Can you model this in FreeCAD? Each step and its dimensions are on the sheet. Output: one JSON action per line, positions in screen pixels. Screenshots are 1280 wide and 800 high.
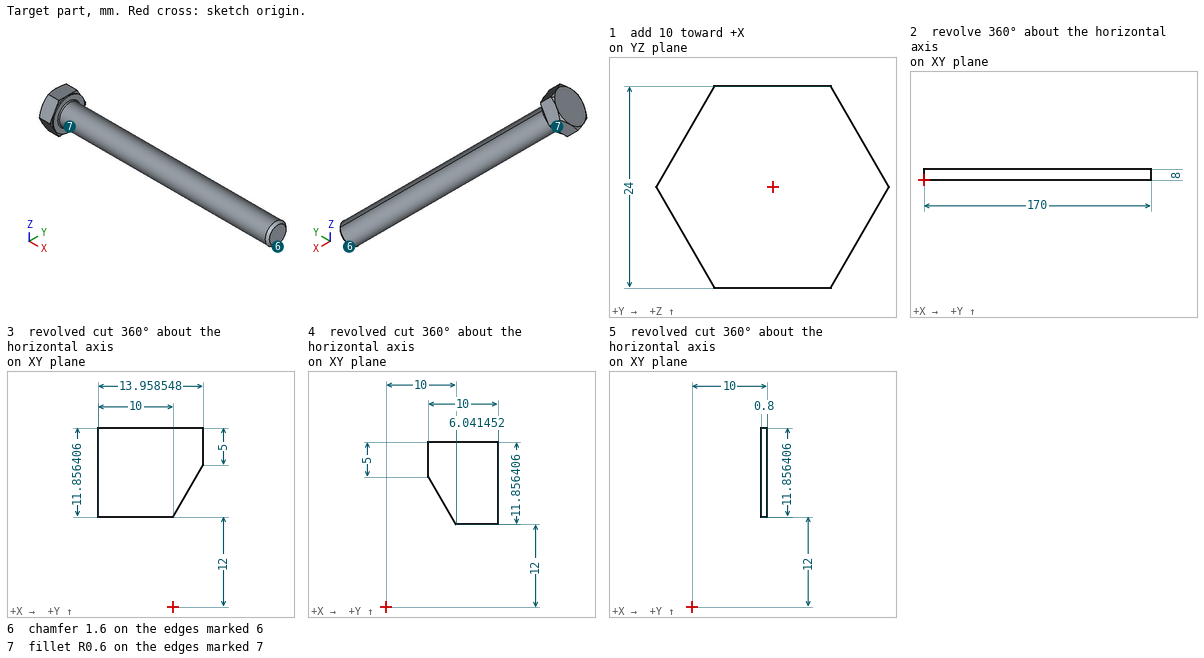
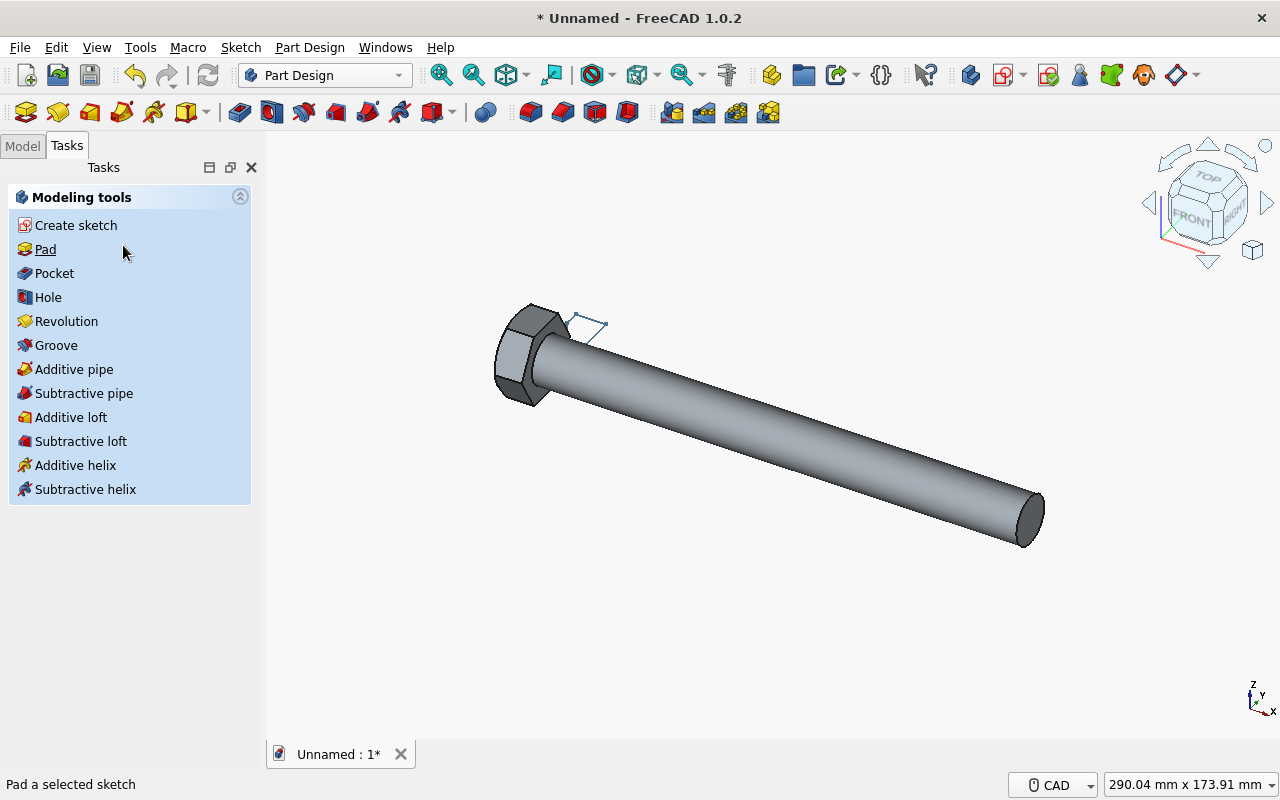
{"action": "left_click", "coordinate": [304, 112]}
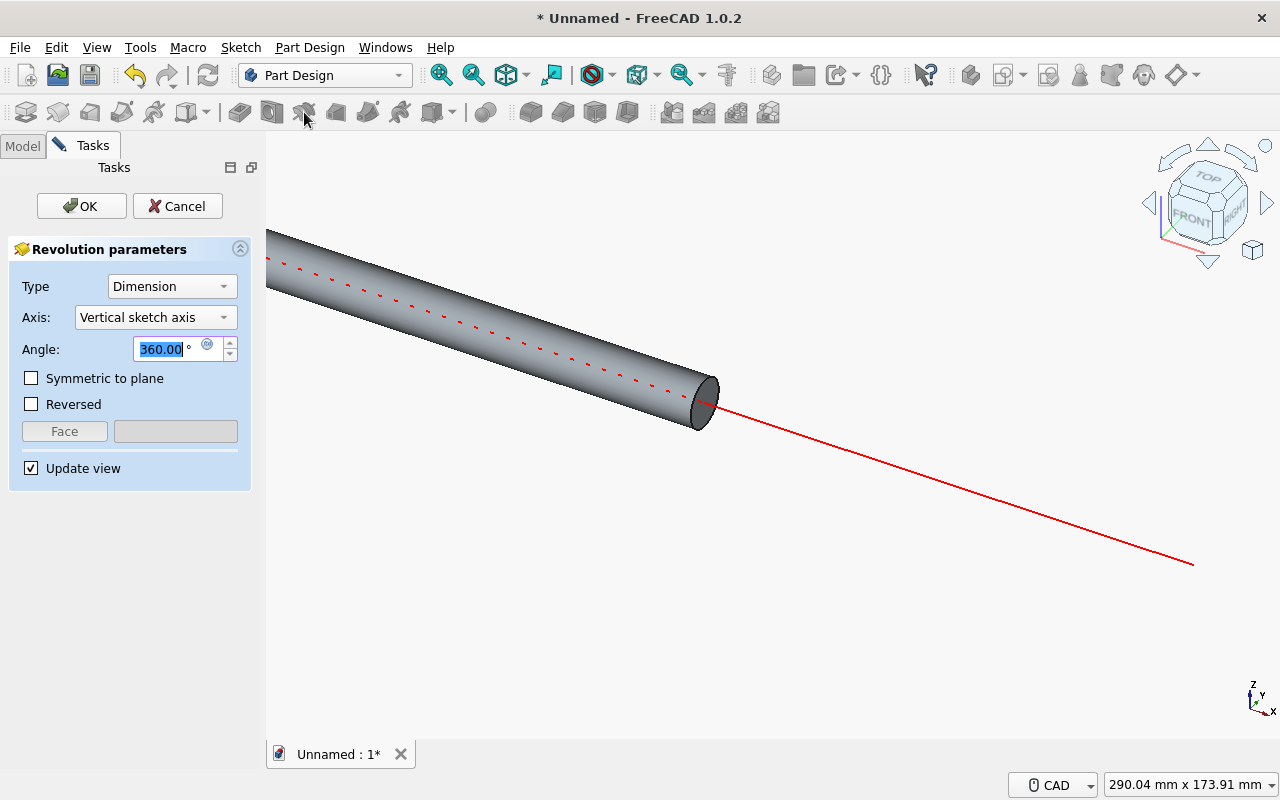
{"action": "left_click", "coordinate": [156, 318]}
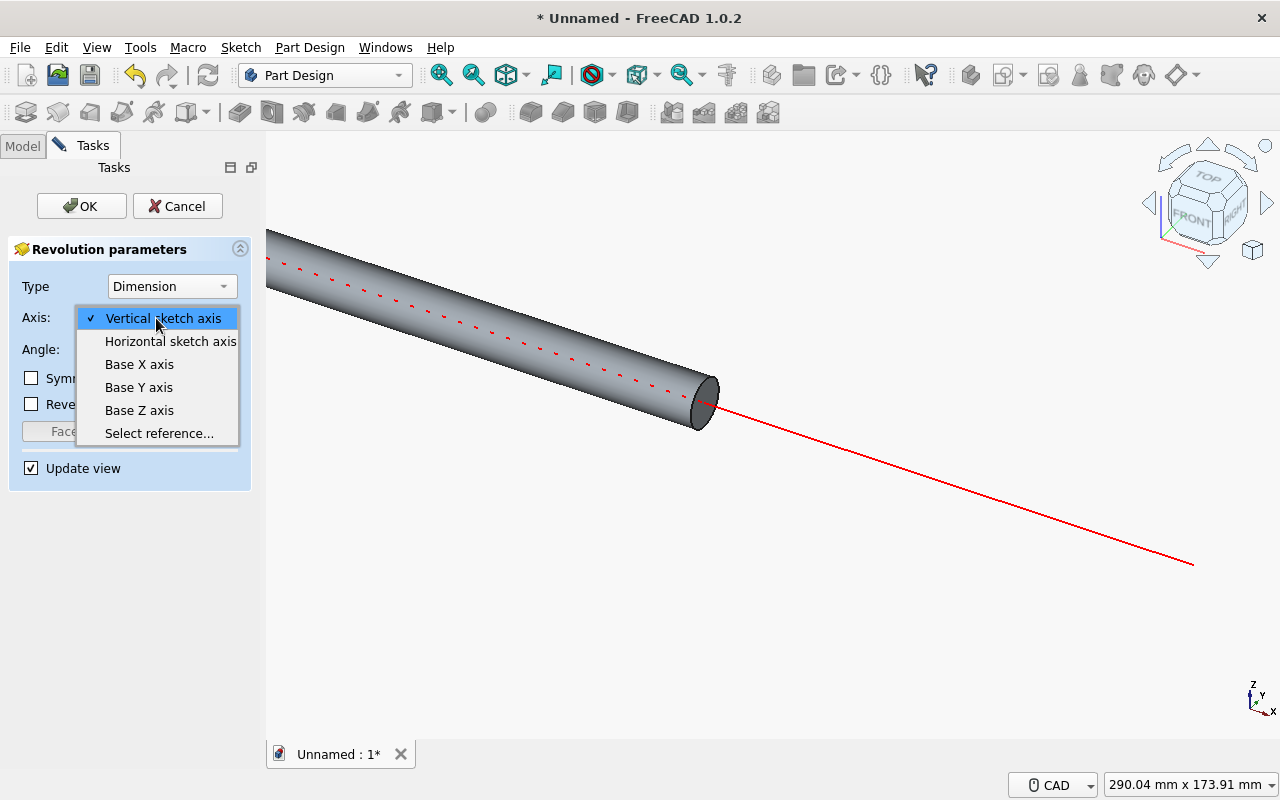
{"action": "left_click", "coordinate": [156, 342]}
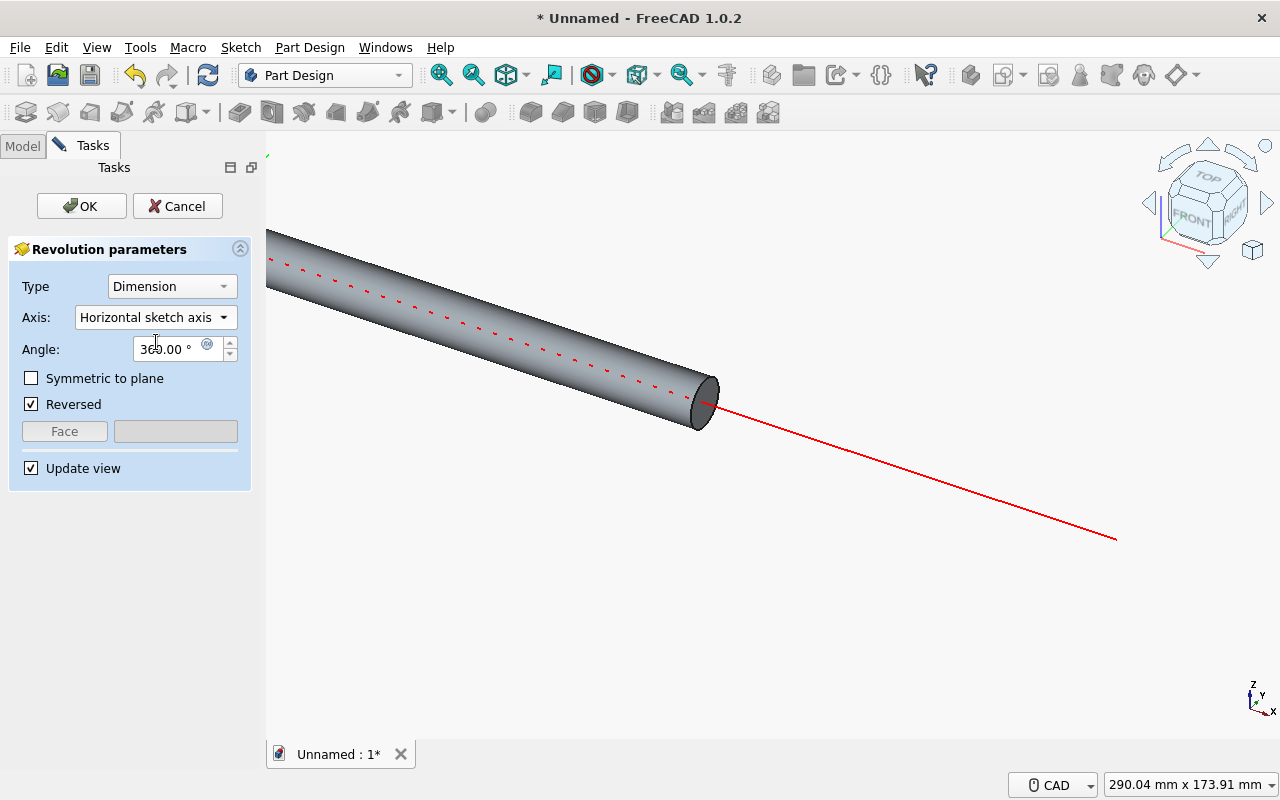
{"action": "left_click", "coordinate": [82, 206]}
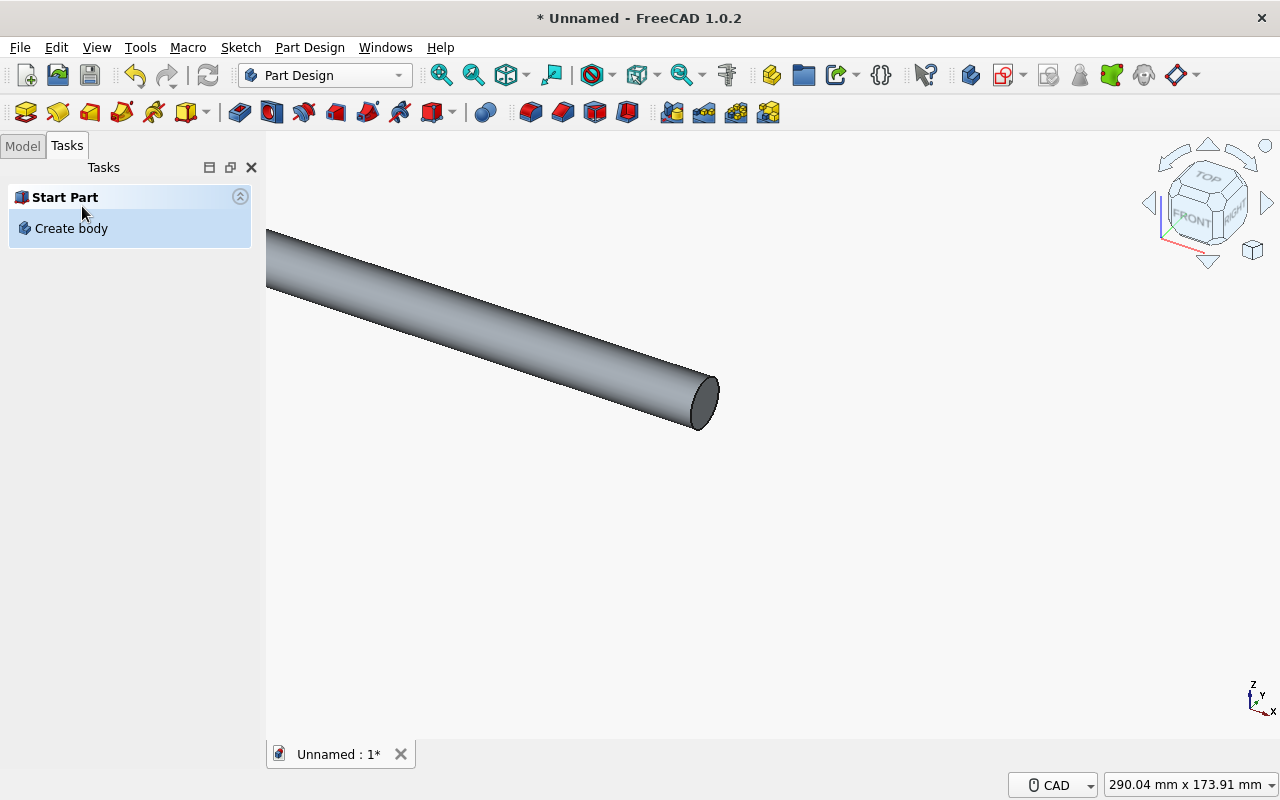
{"action": "left_click", "coordinate": [442, 76]}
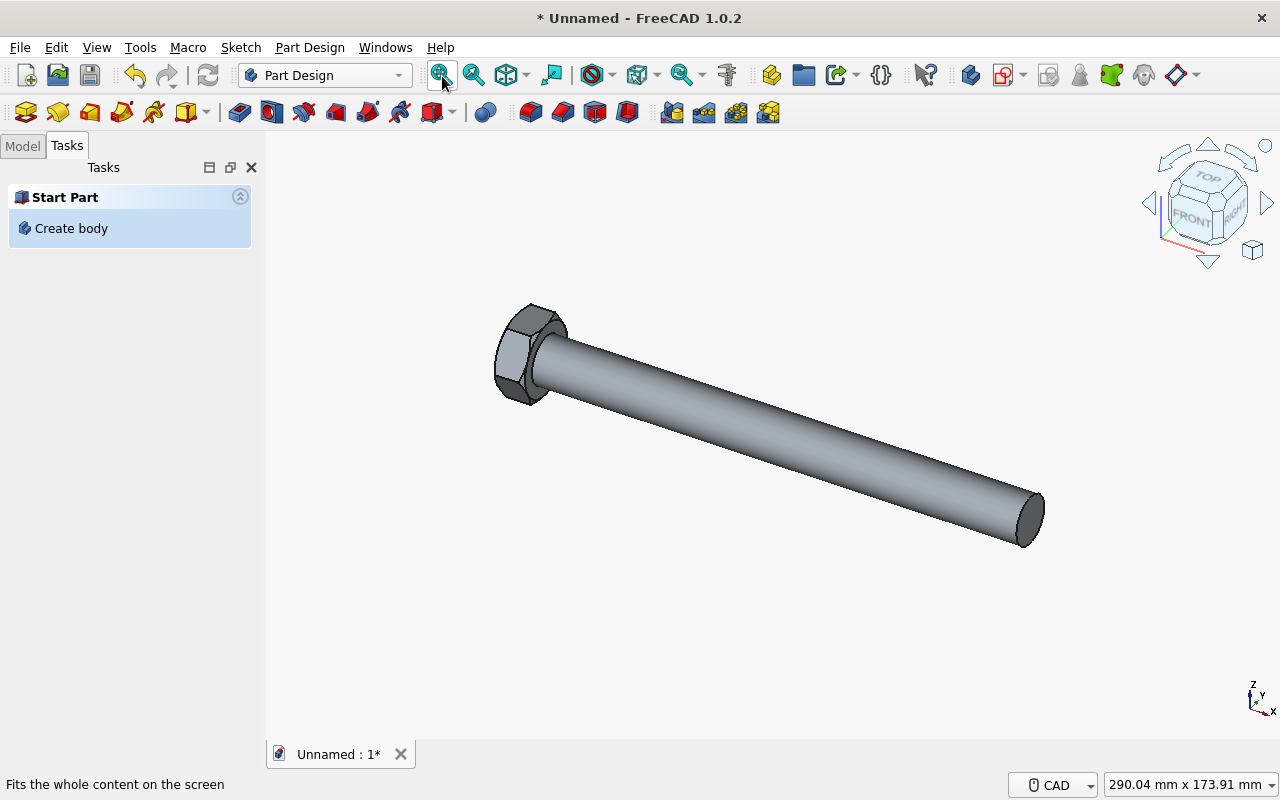
{"action": "left_click", "coordinate": [1004, 76]}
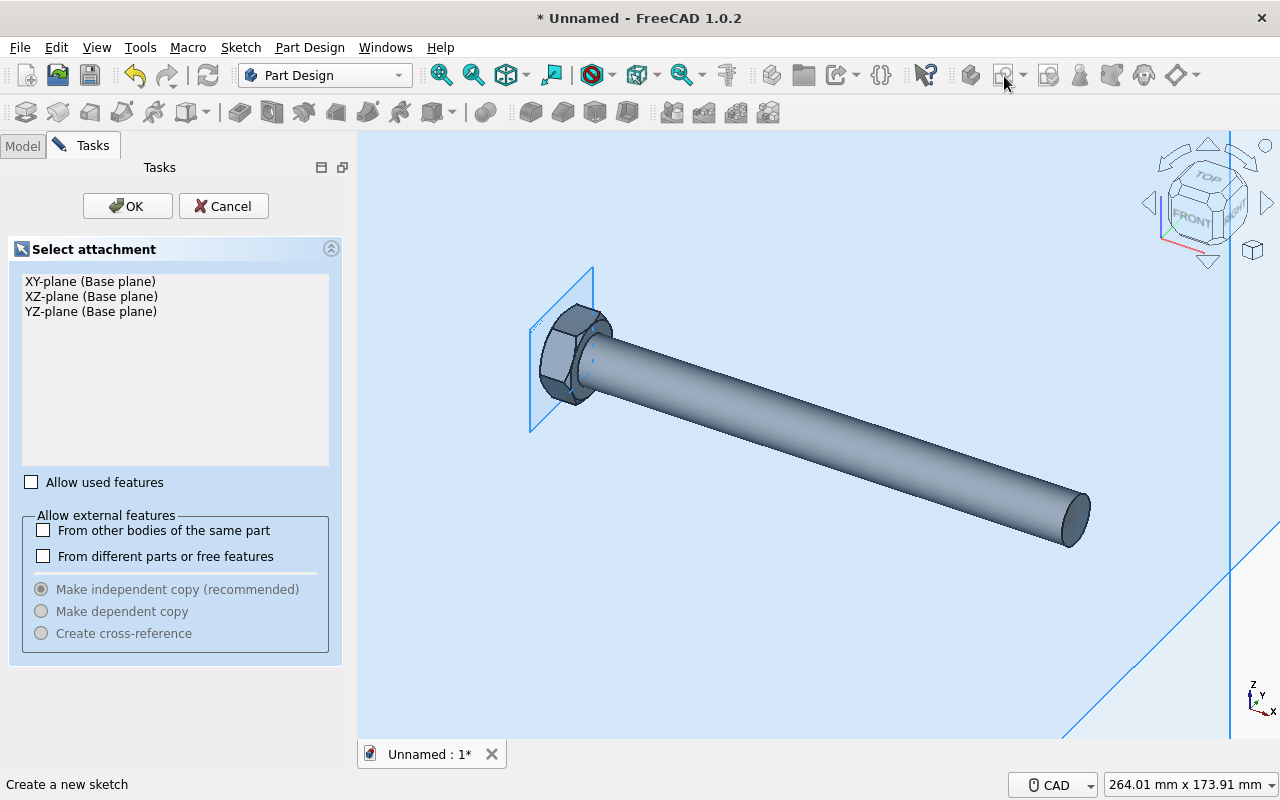
{"action": "left_click", "coordinate": [82, 282]}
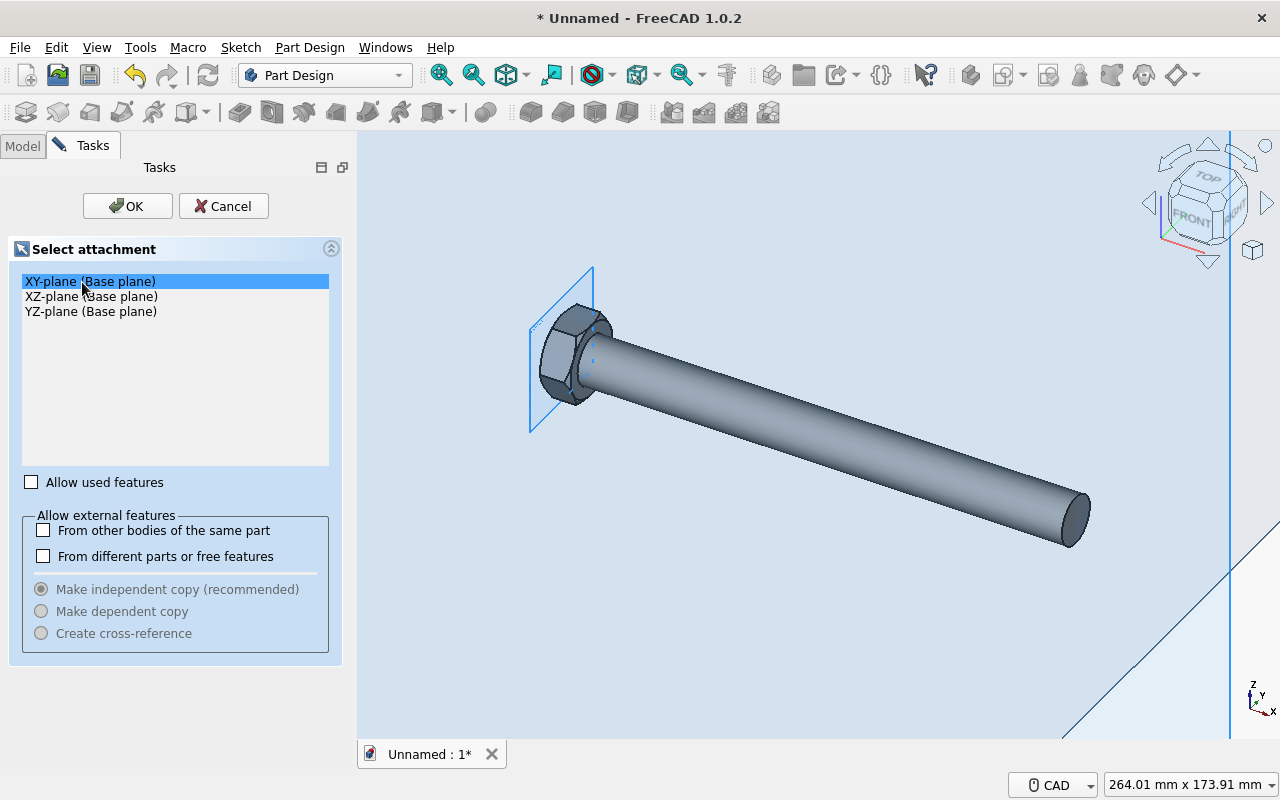
{"action": "left_click", "coordinate": [128, 206]}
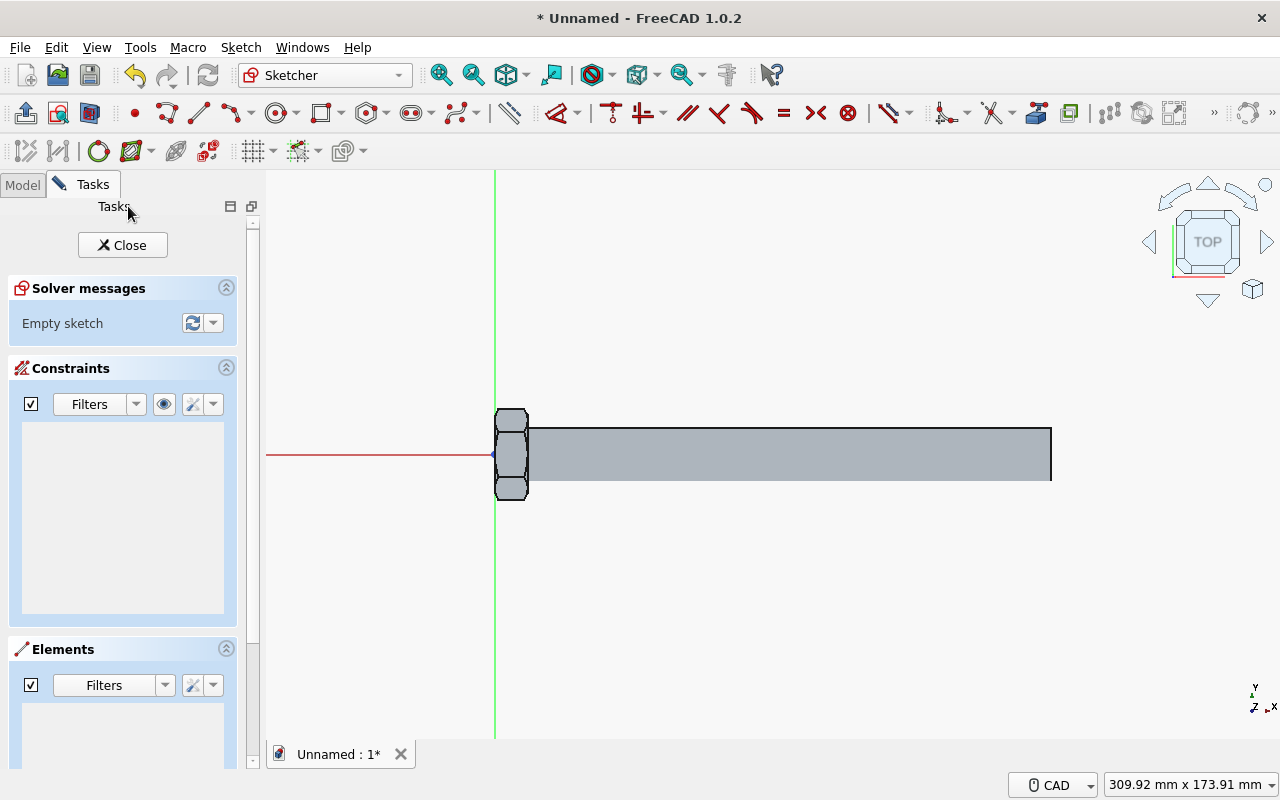
{"action": "key", "text": "q s"}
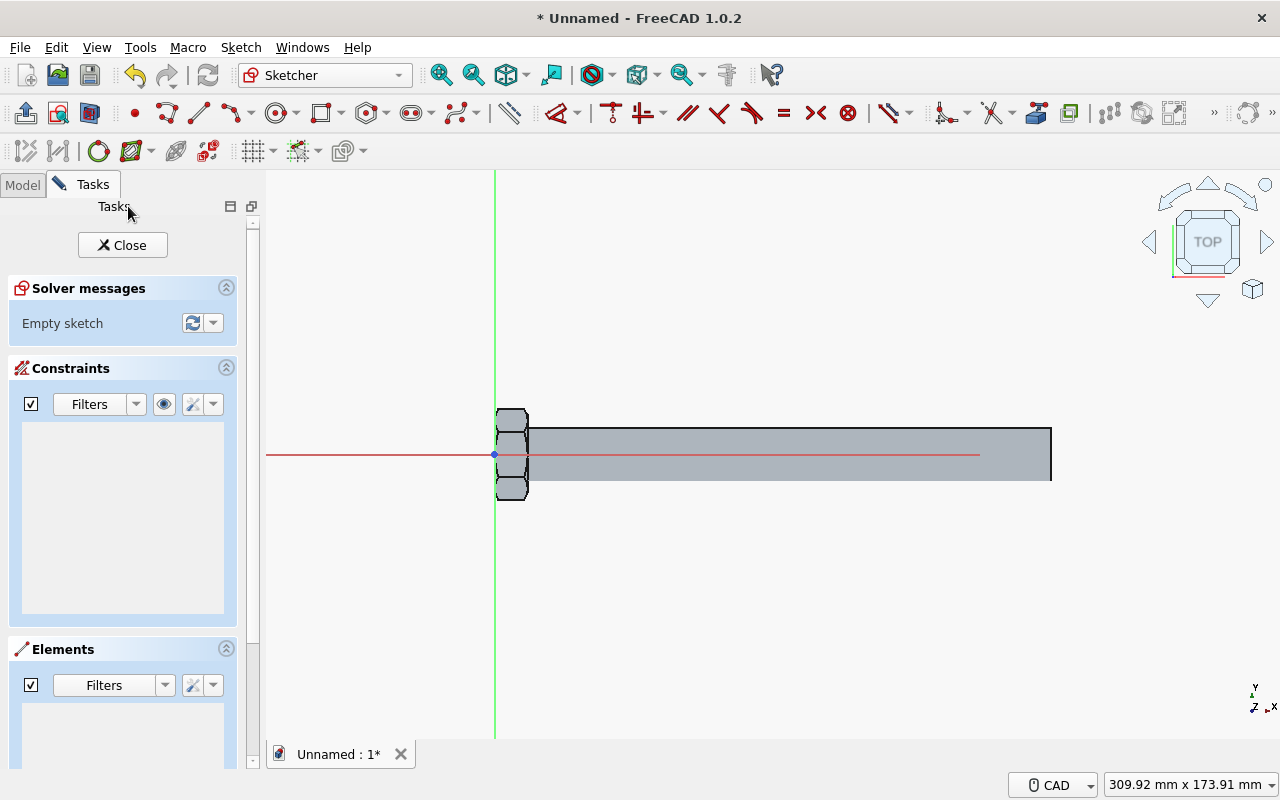
{"action": "scroll", "coordinate": [462, 406], "scroll_direction": "up", "scroll_amount": 8}